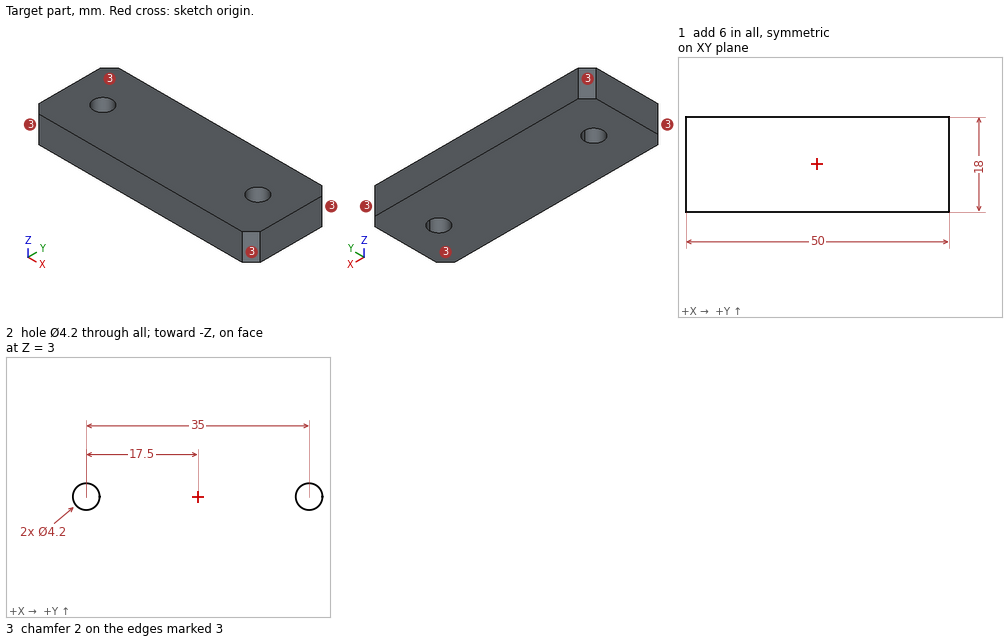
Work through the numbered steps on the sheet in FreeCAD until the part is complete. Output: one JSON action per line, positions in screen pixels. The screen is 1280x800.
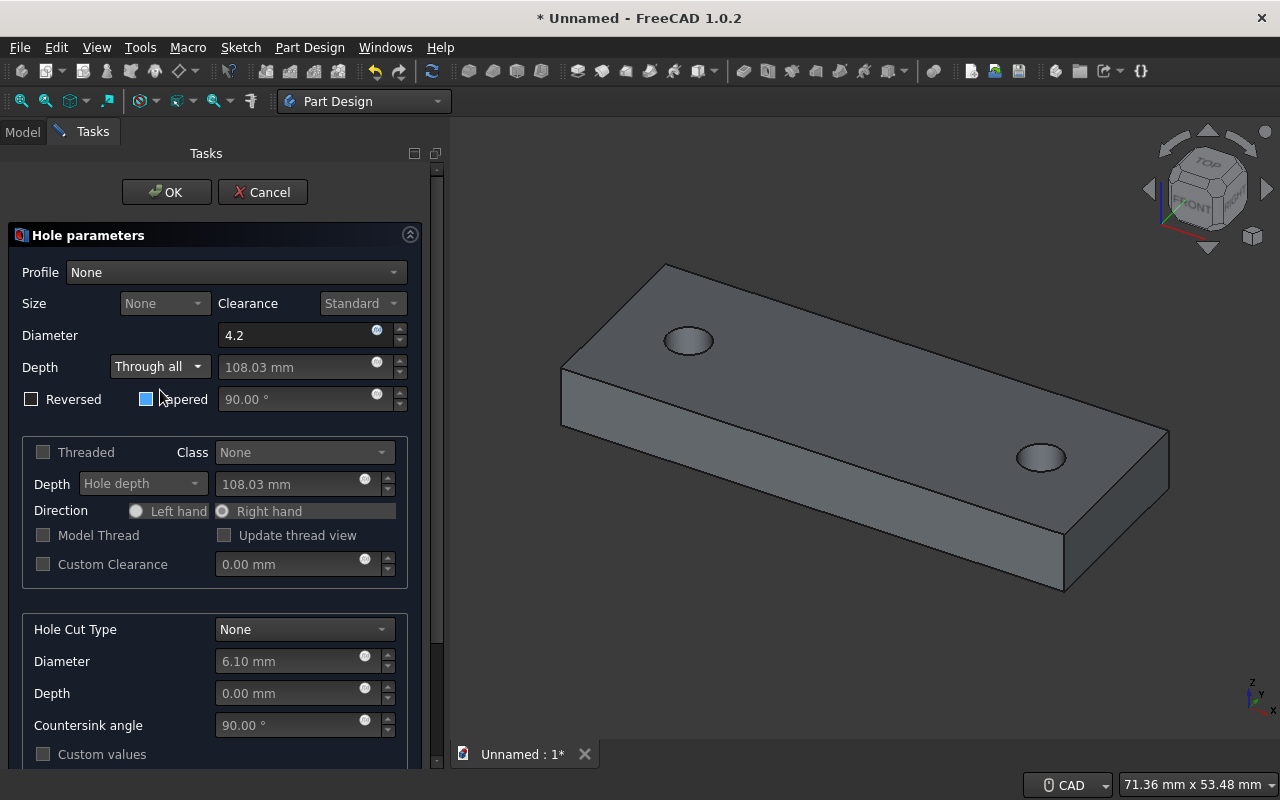
{"action": "left_click", "coordinate": [167, 192]}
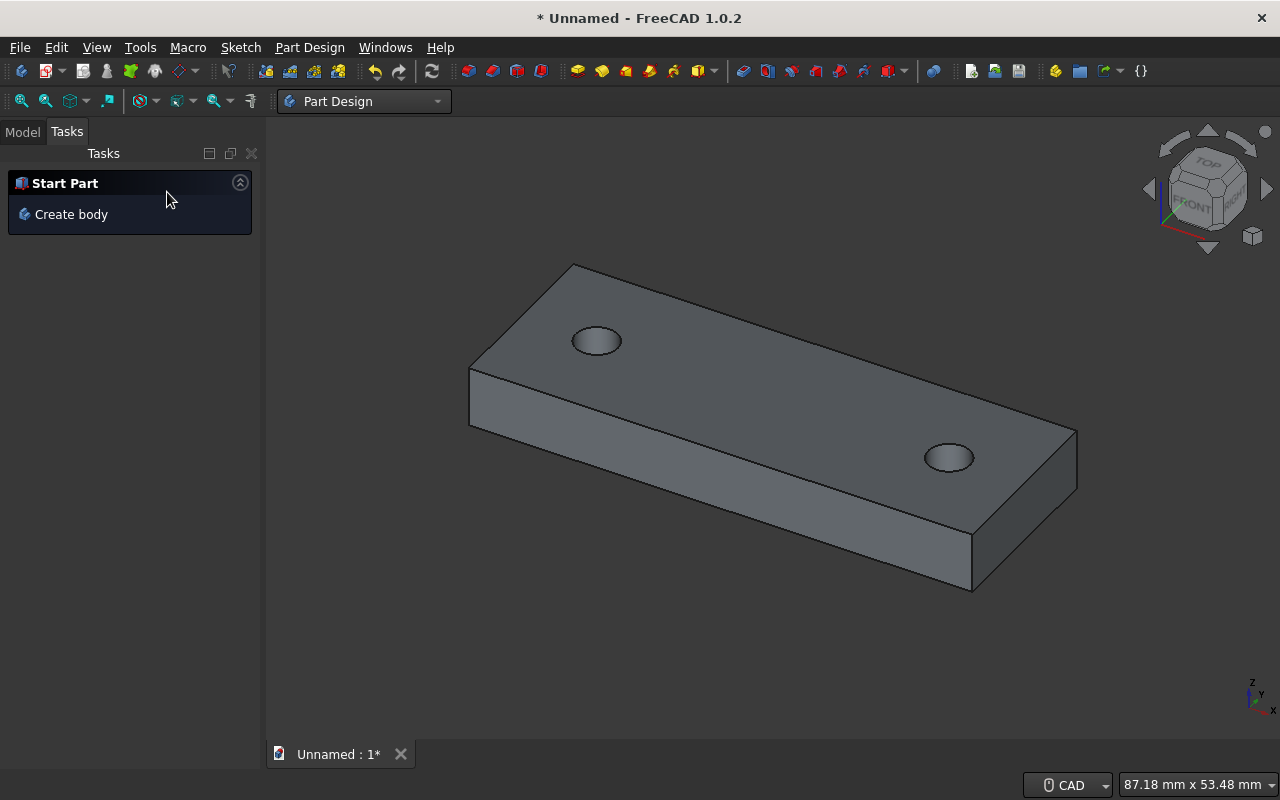
{"action": "left_click", "coordinate": [972, 562]}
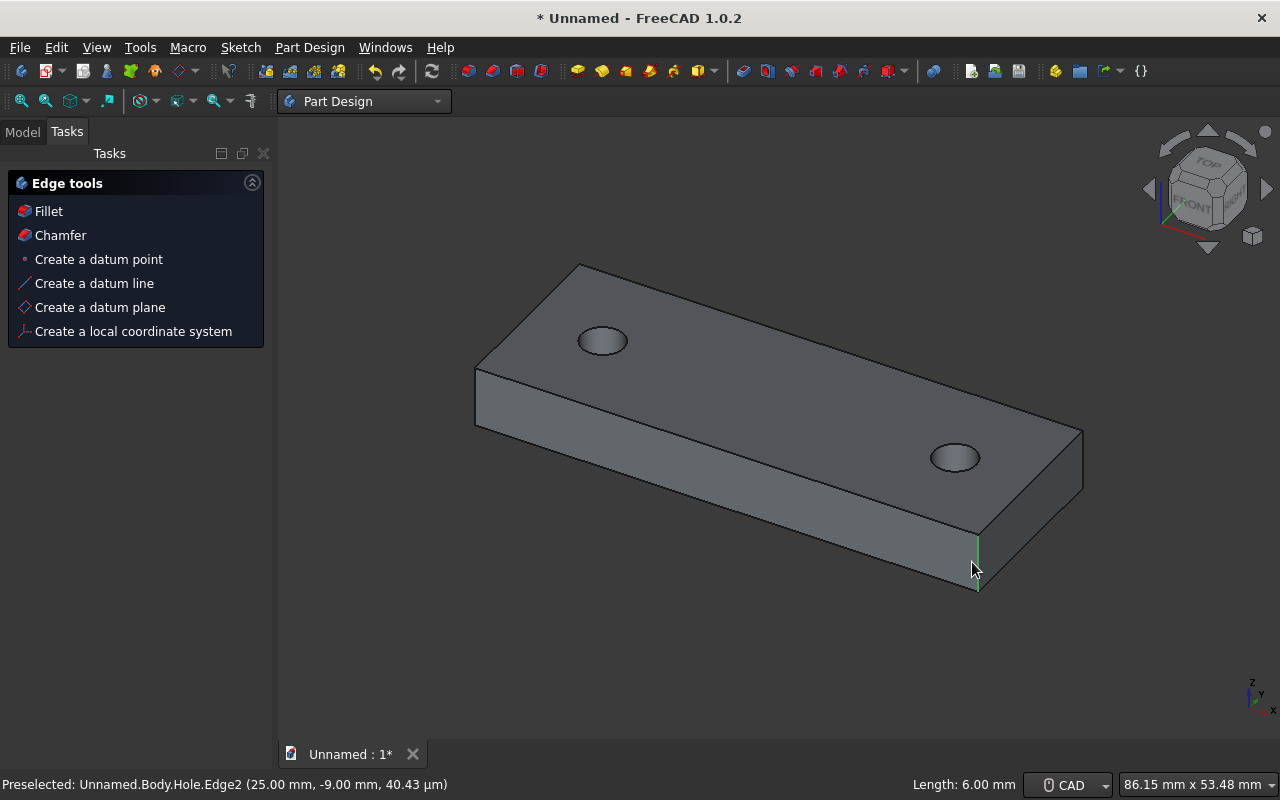
{"action": "key", "text": "0"}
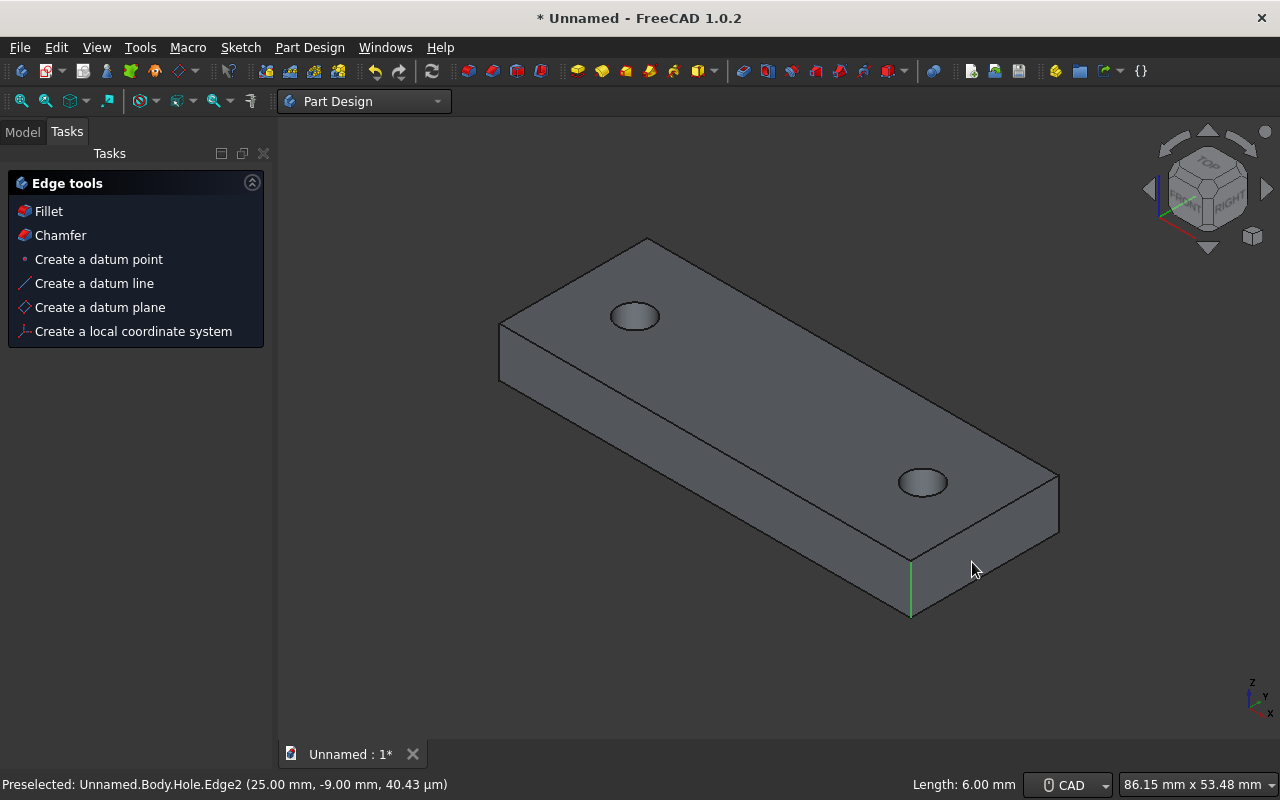
{"action": "key", "text": "2"}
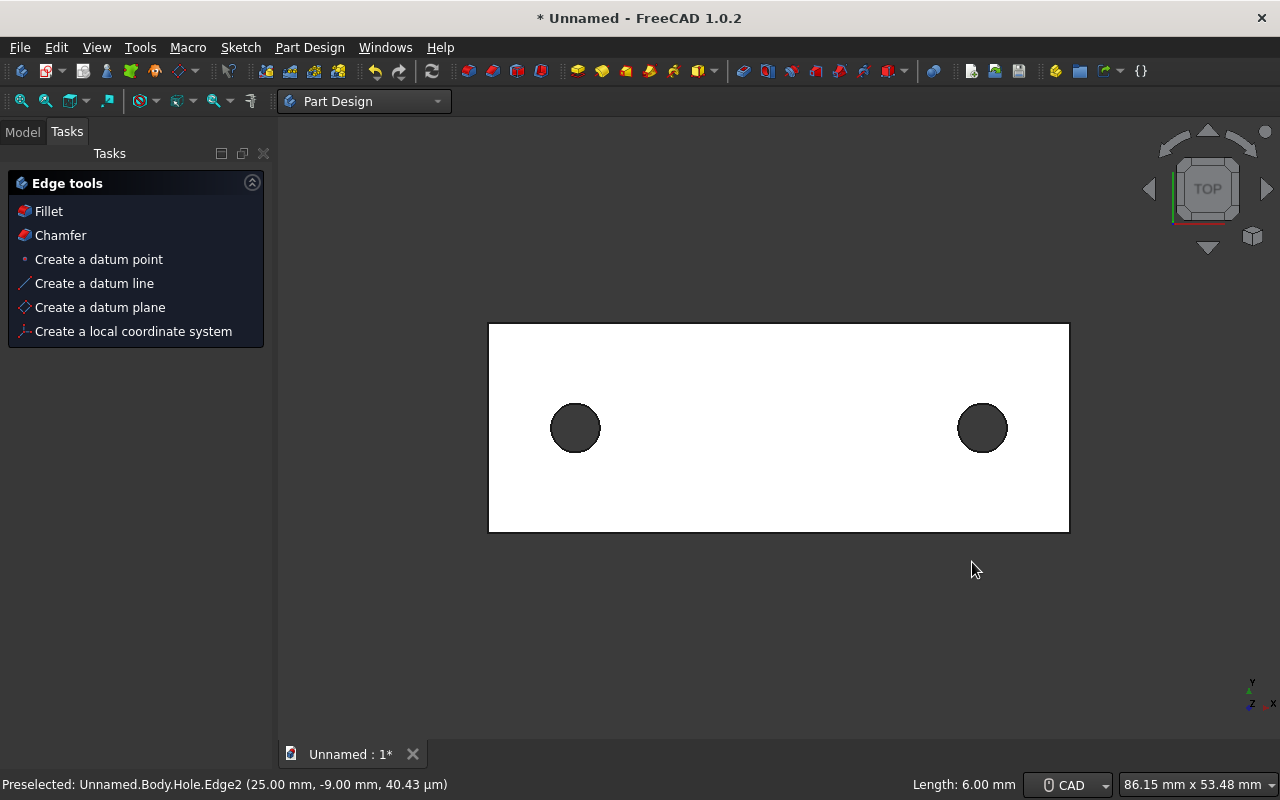
{"action": "key", "text": "1"}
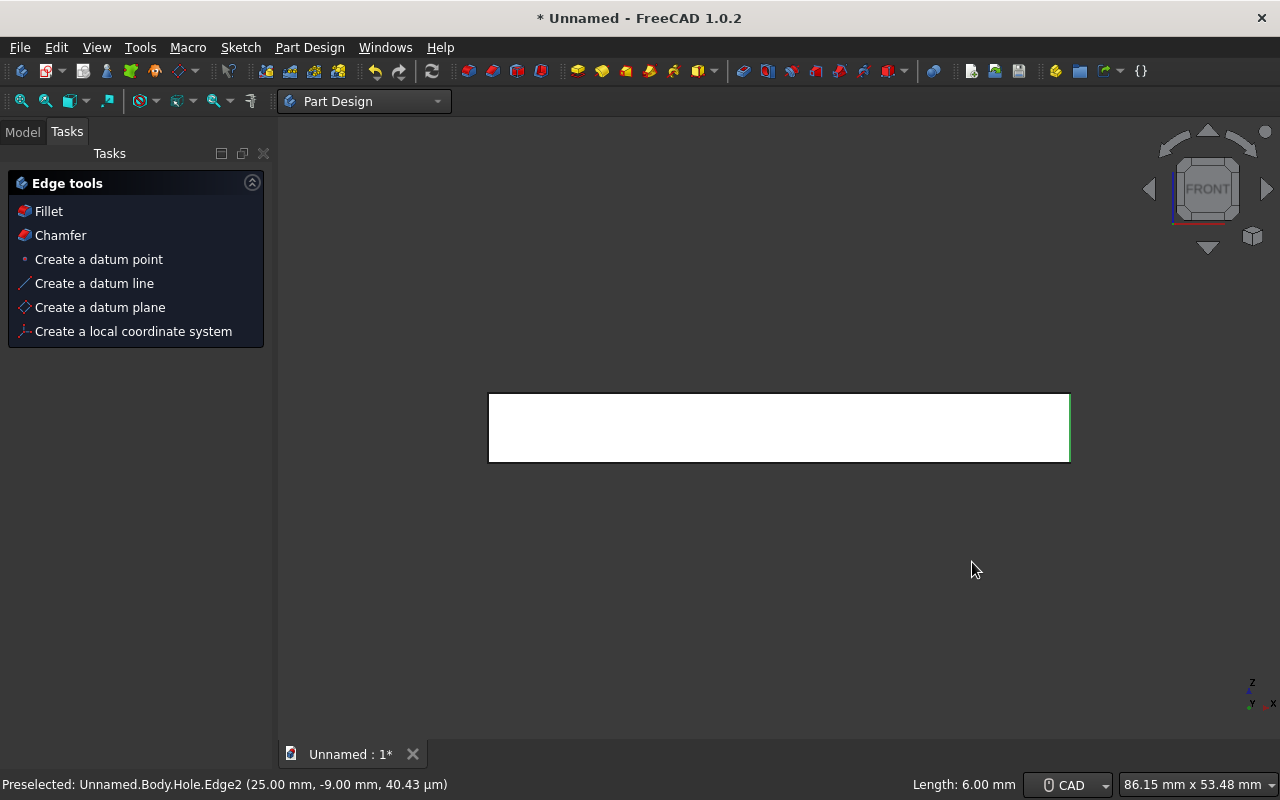
{"action": "left_click", "coordinate": [488, 427], "text": "ctrl"}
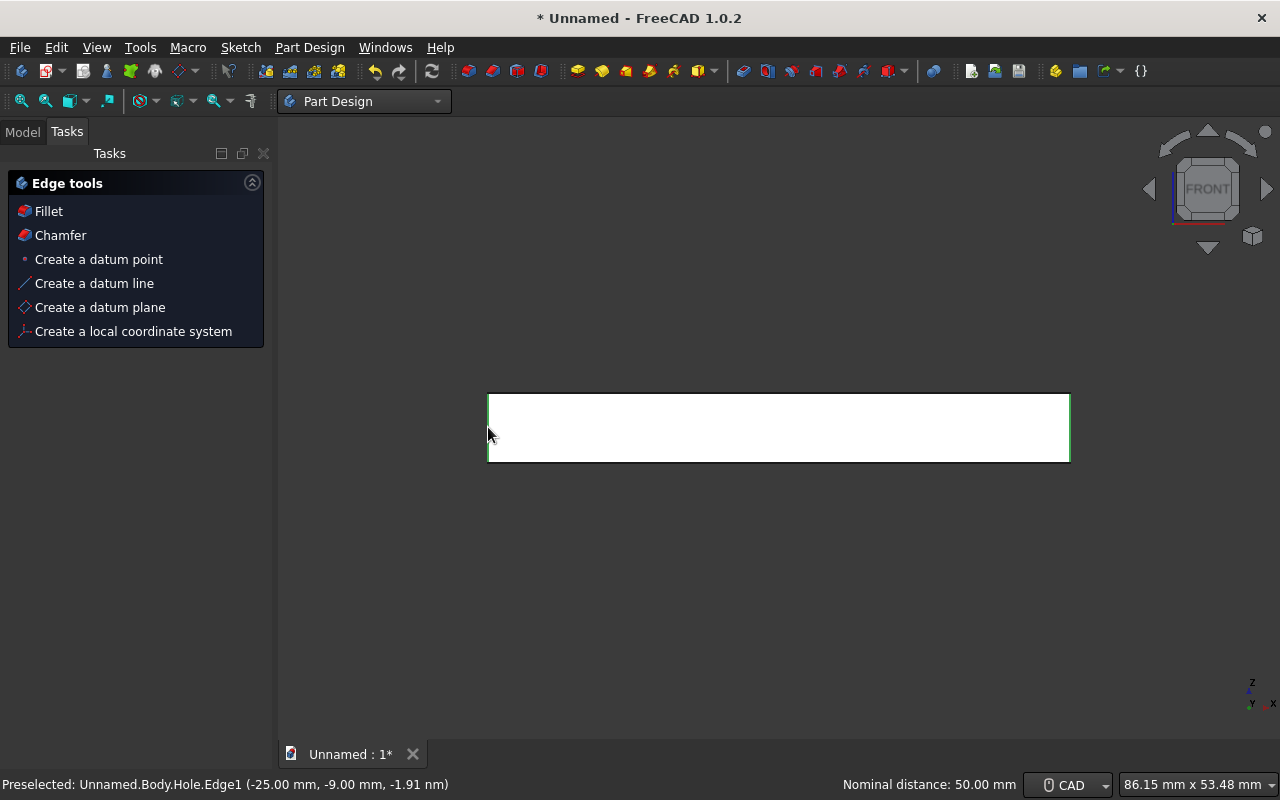
{"action": "key", "text": "3"}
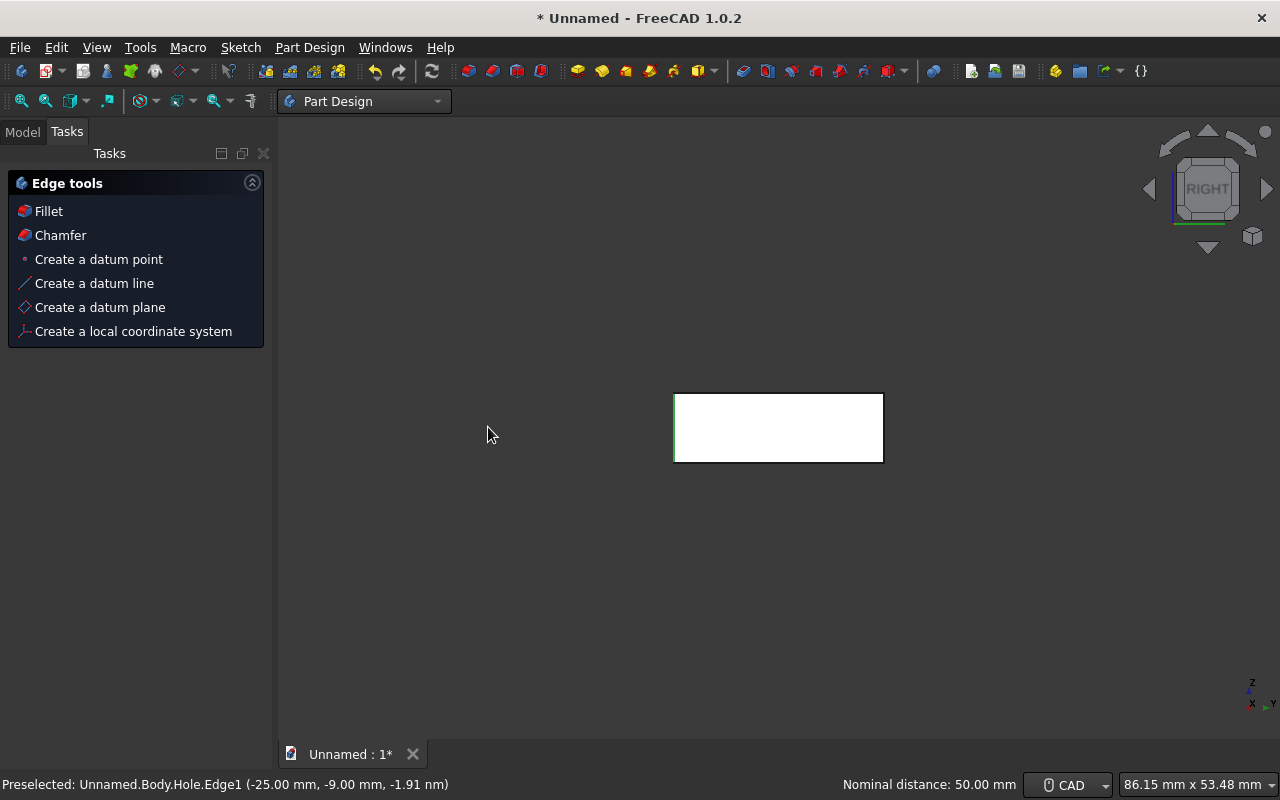
{"action": "key", "text": "v f"}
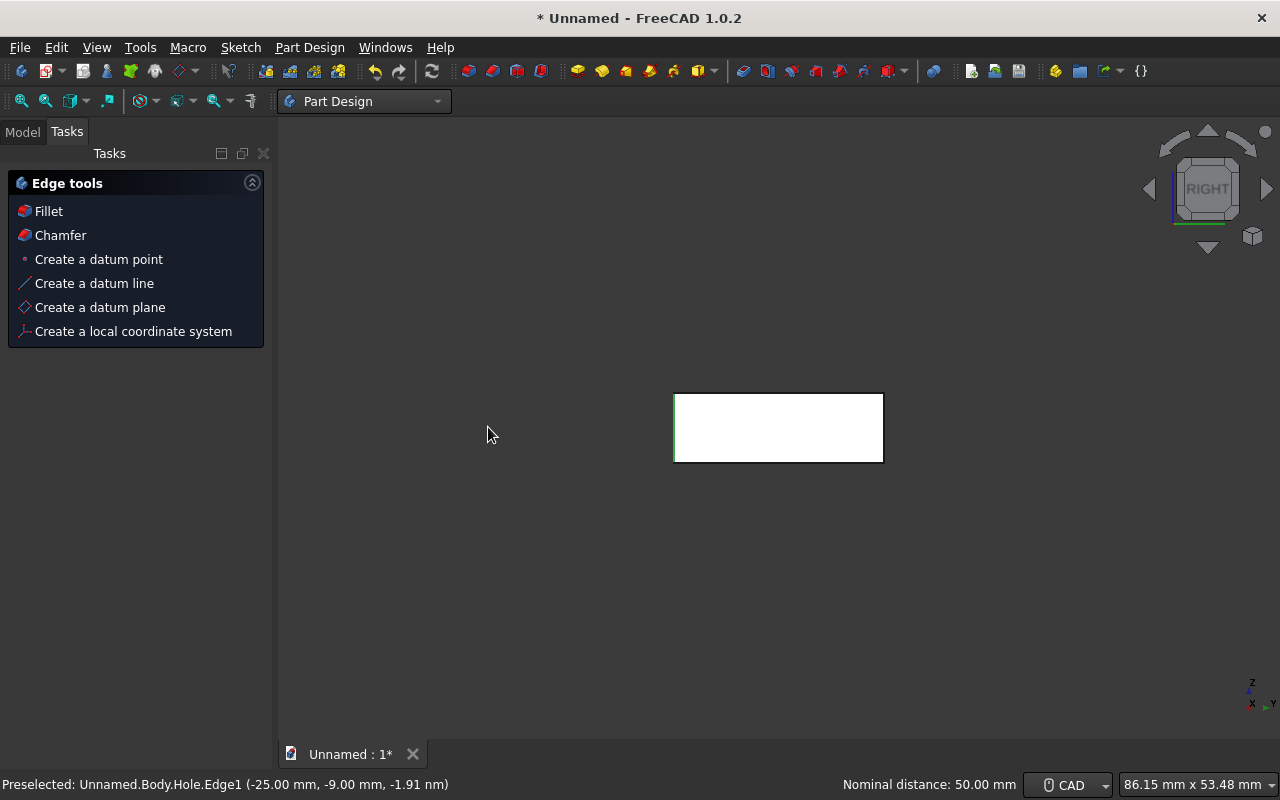
{"action": "left_click", "coordinate": [884, 427], "text": "ctrl"}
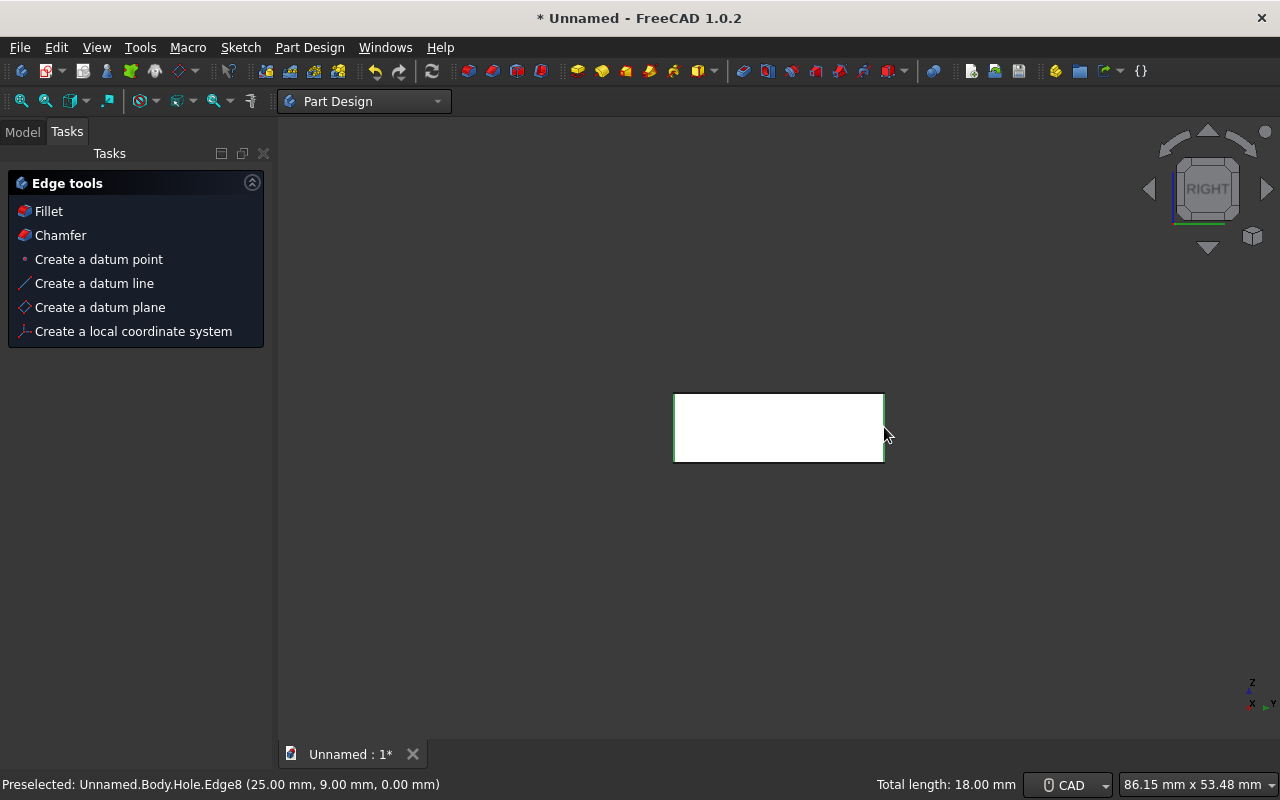
{"action": "key", "text": "5"}